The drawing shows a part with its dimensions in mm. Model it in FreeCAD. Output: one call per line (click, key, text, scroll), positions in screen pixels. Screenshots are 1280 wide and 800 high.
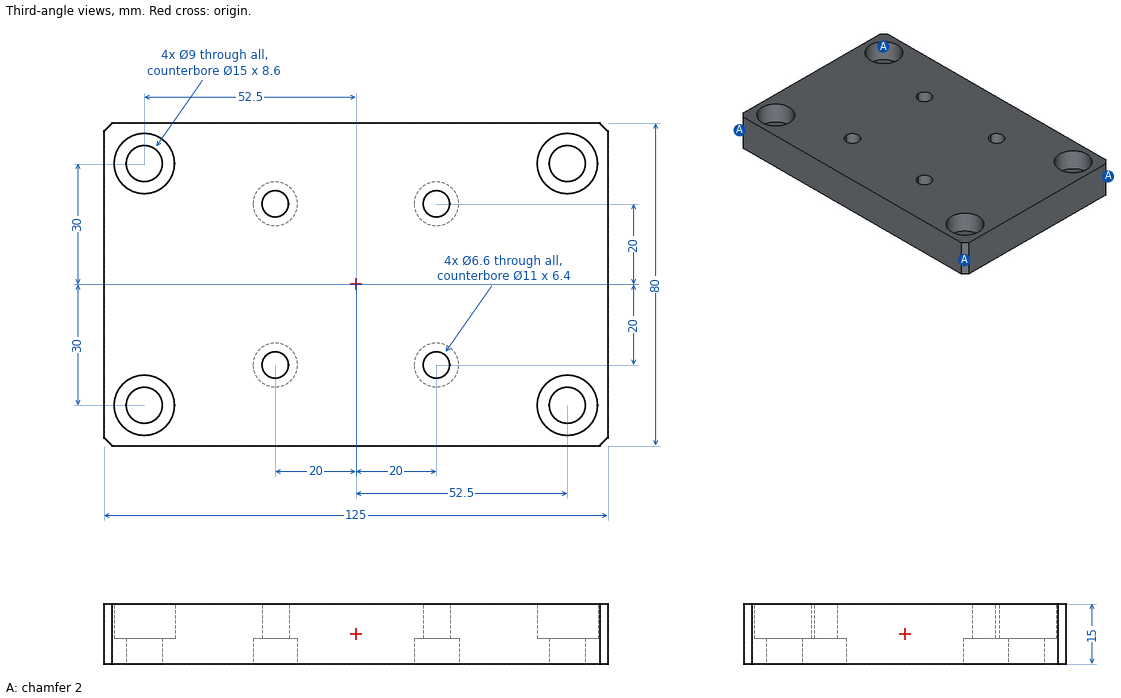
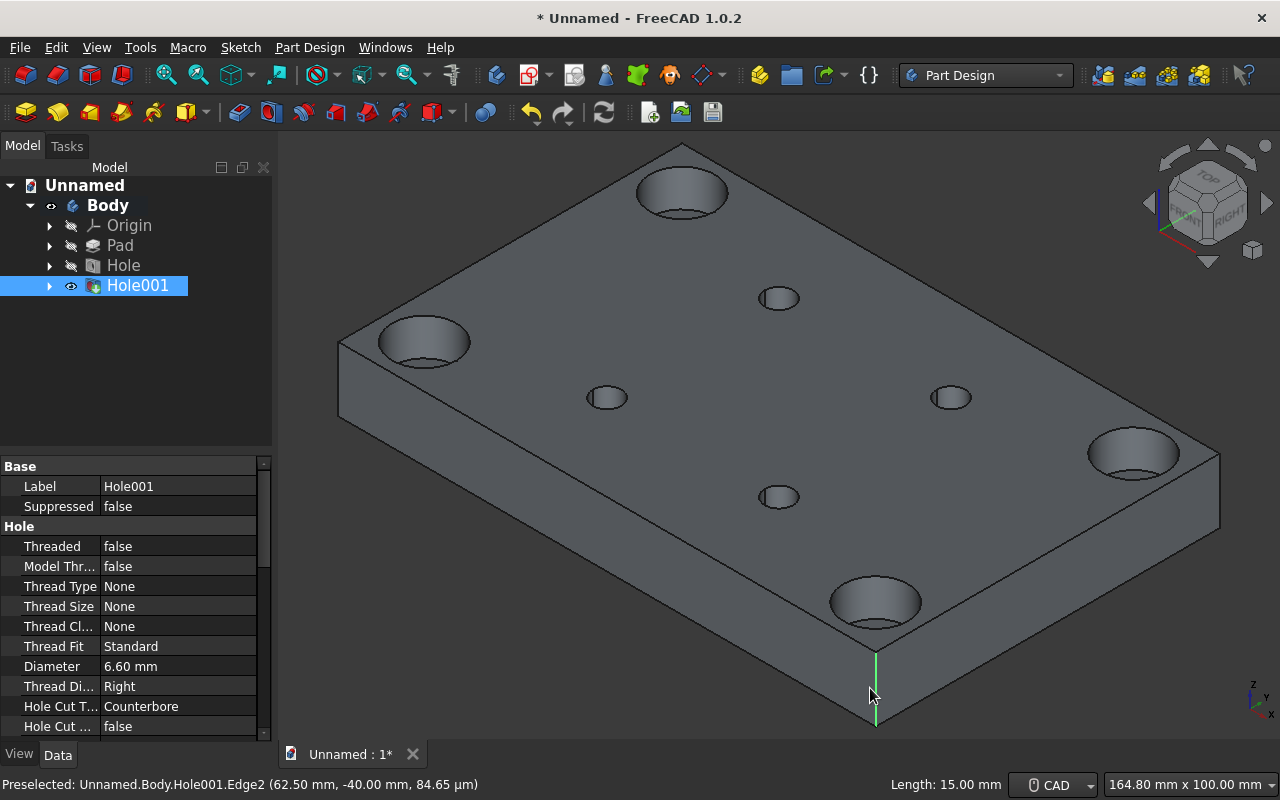
key(2)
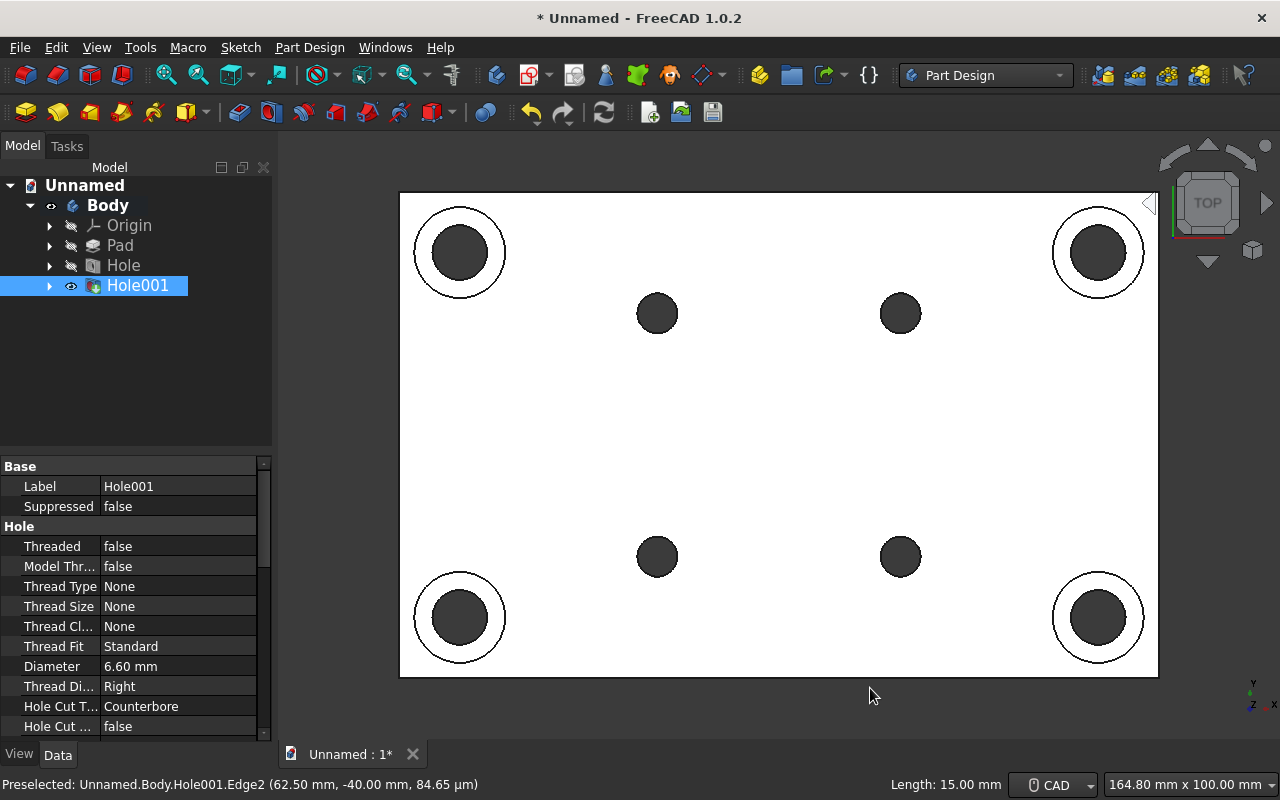
key(1)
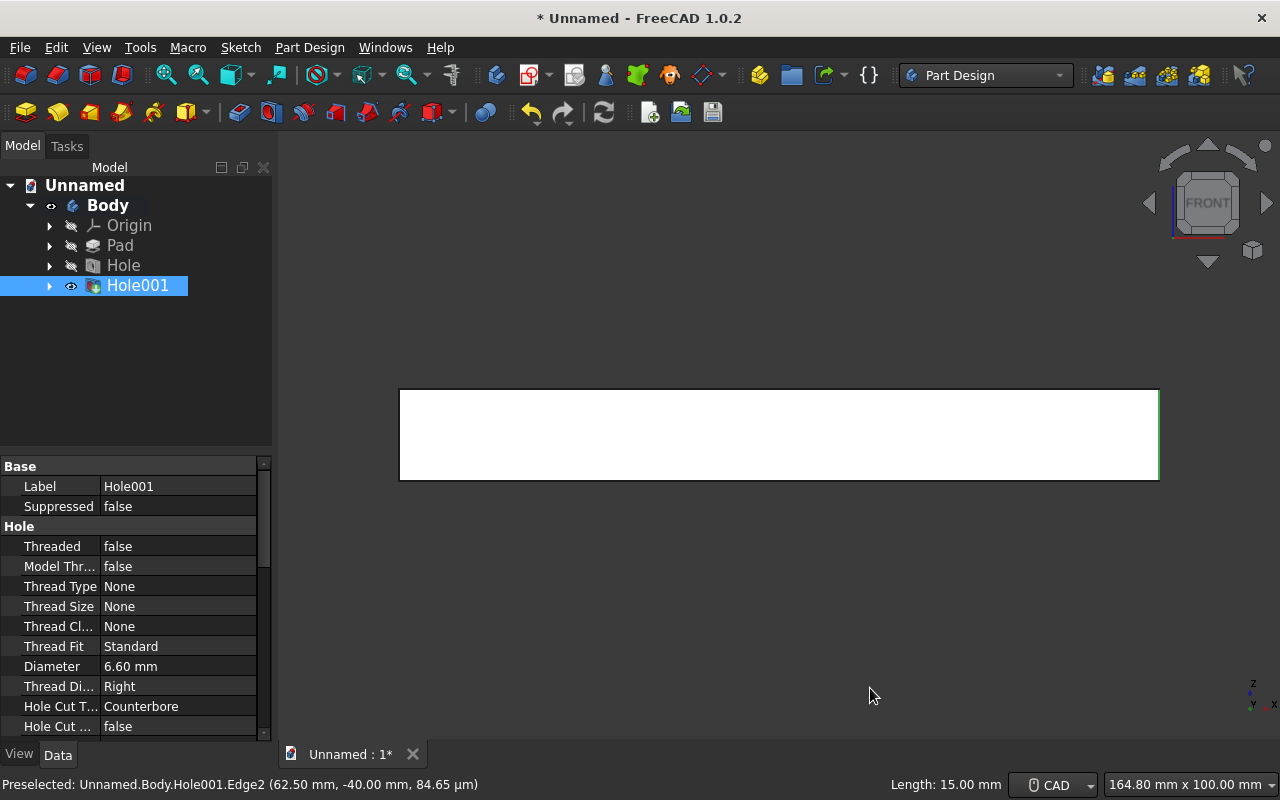
click(399, 434, ctrl)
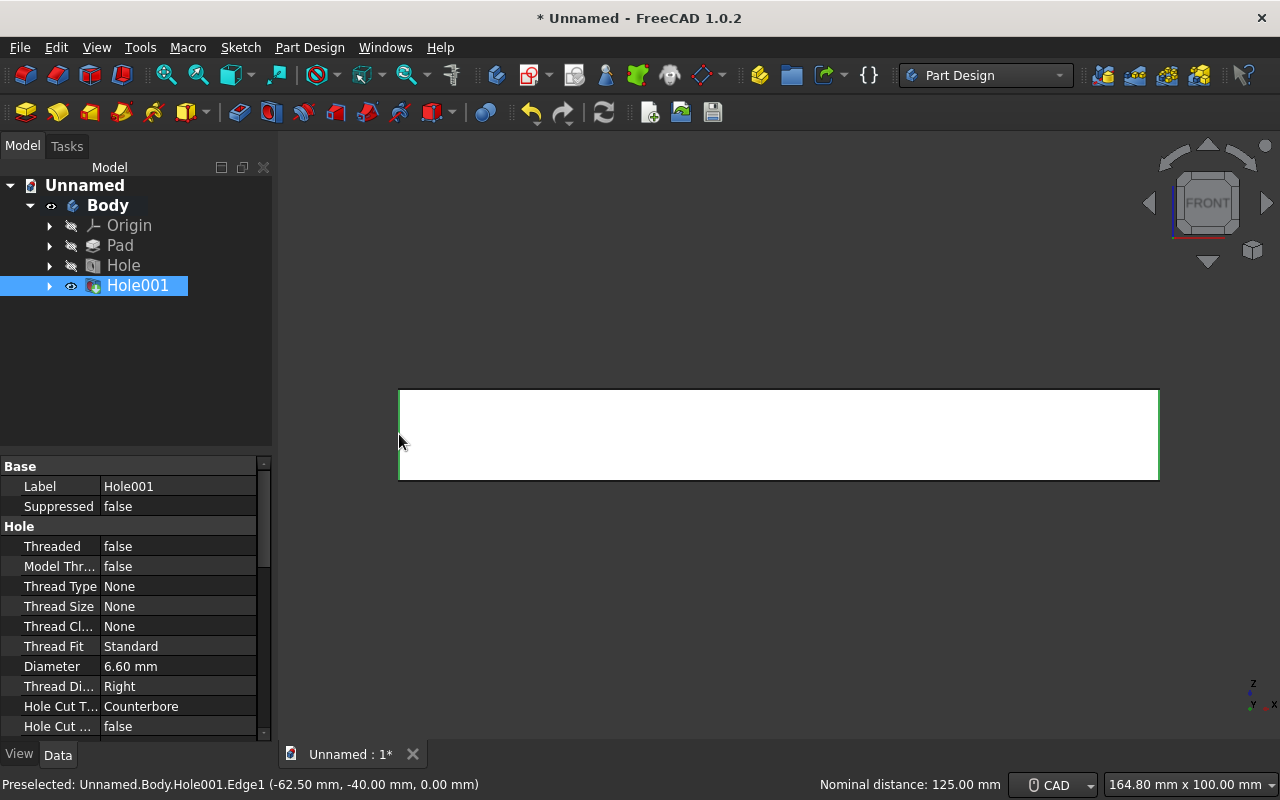
key(3)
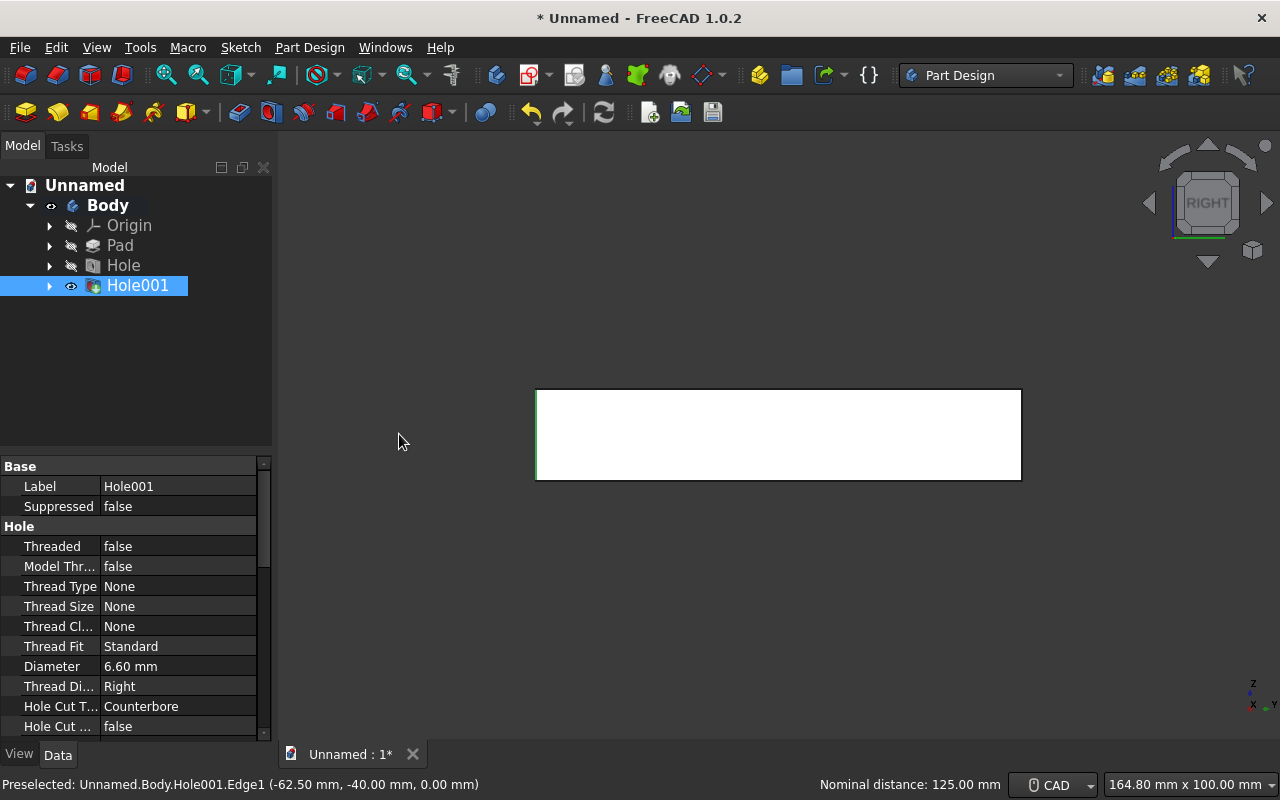
click(1022, 434, ctrl)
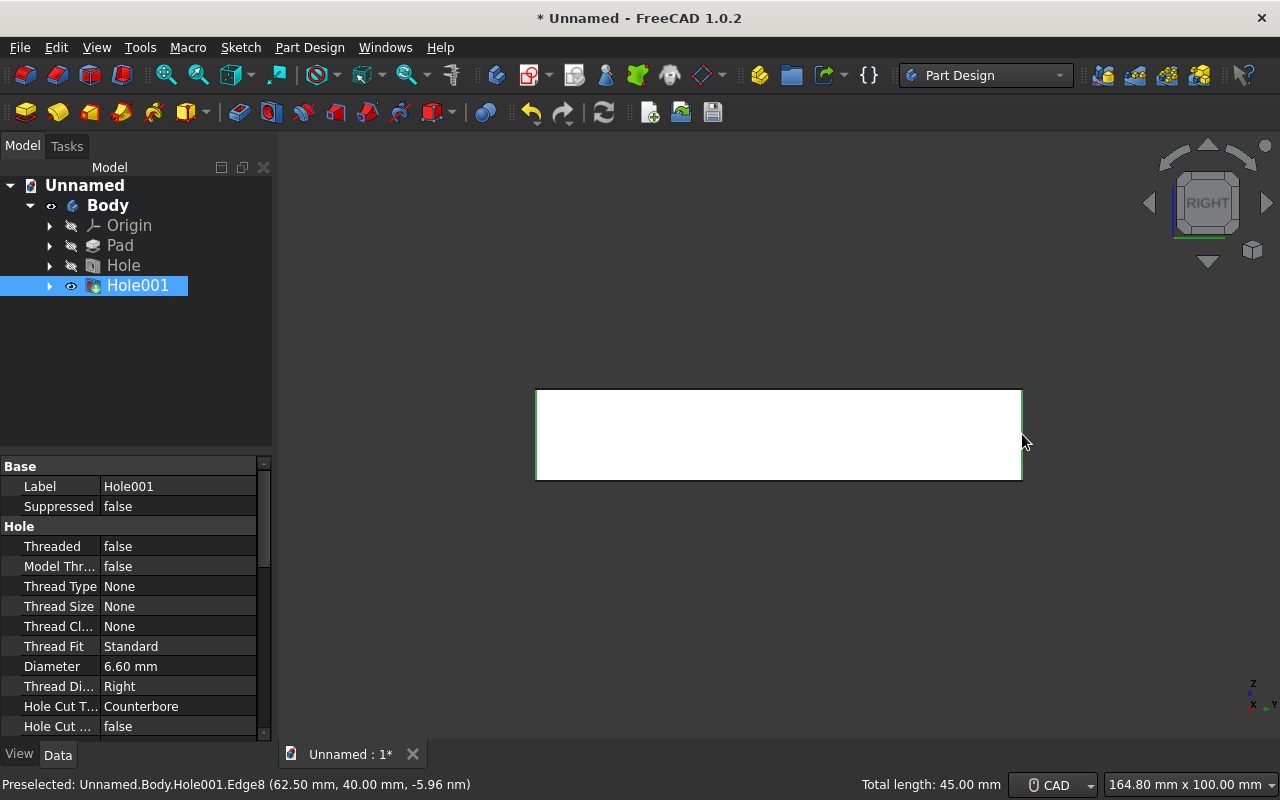
key(5)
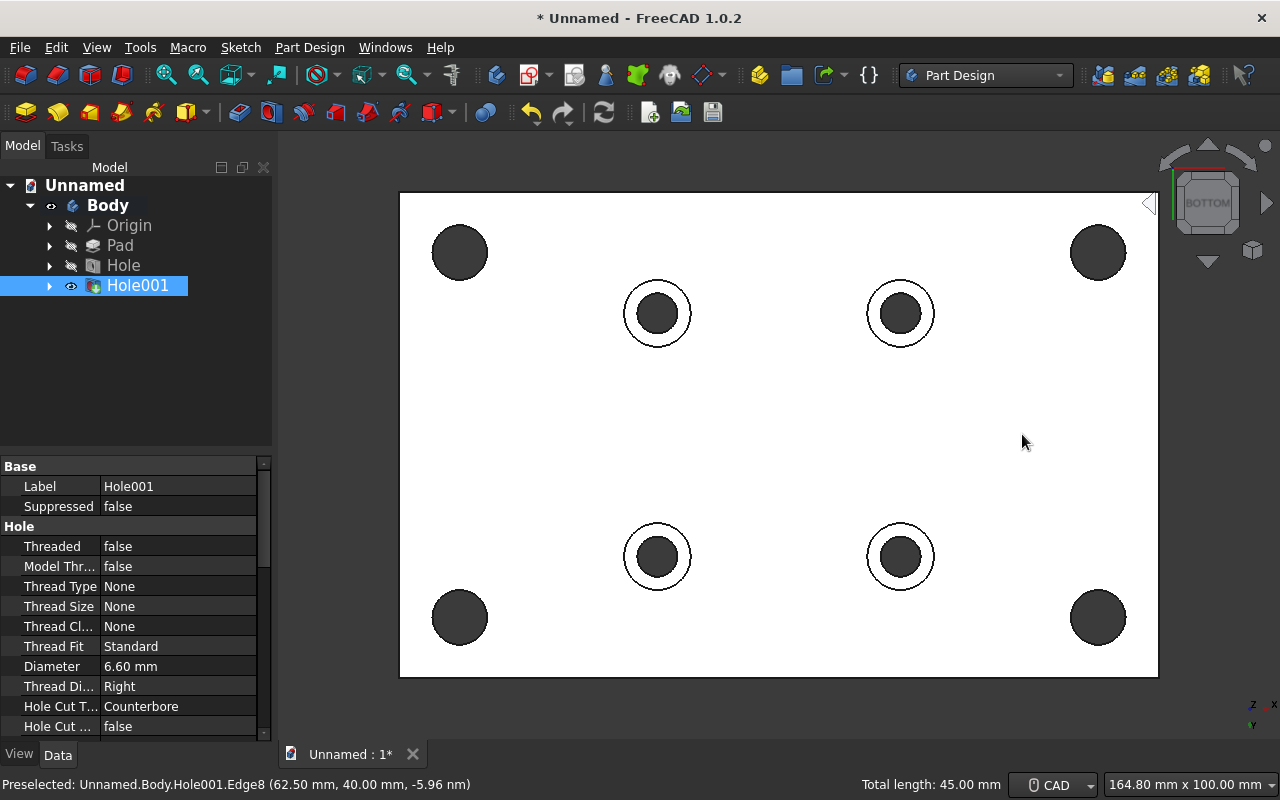
key(4)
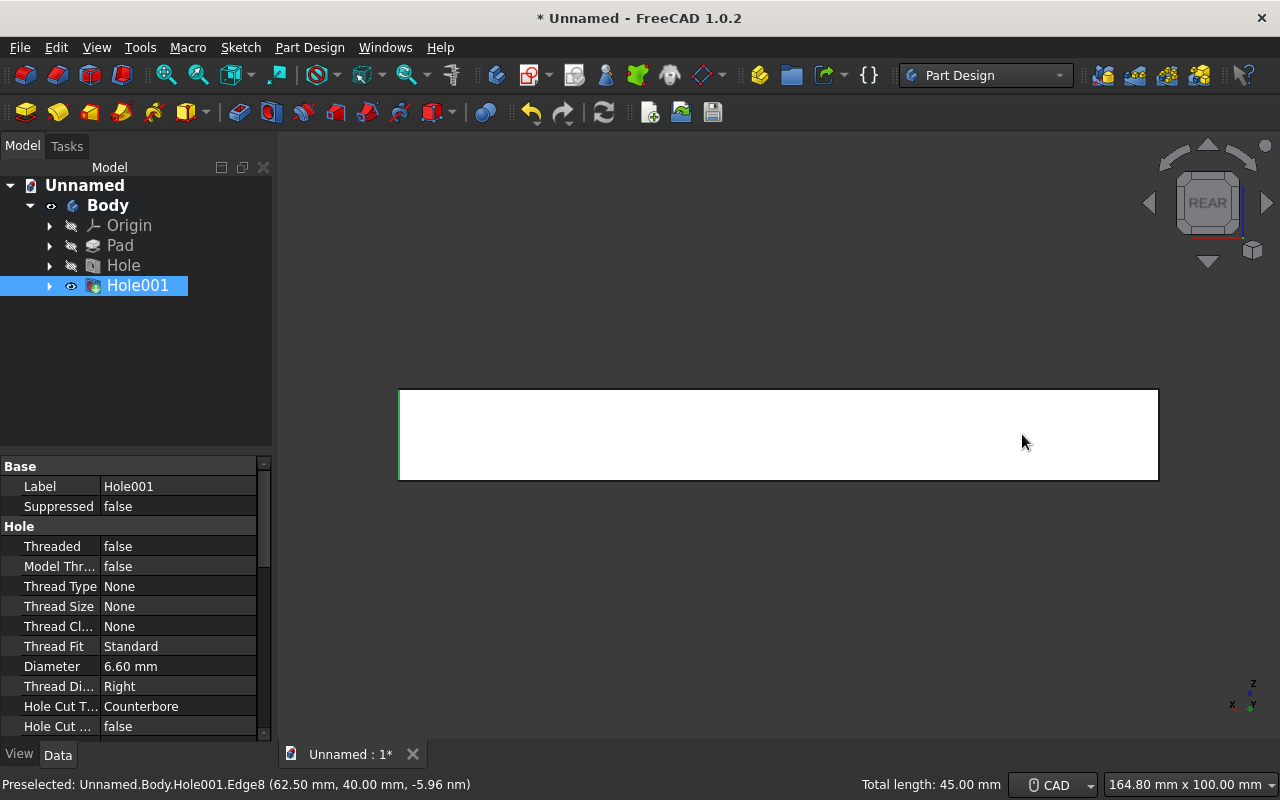
click(1159, 434, ctrl)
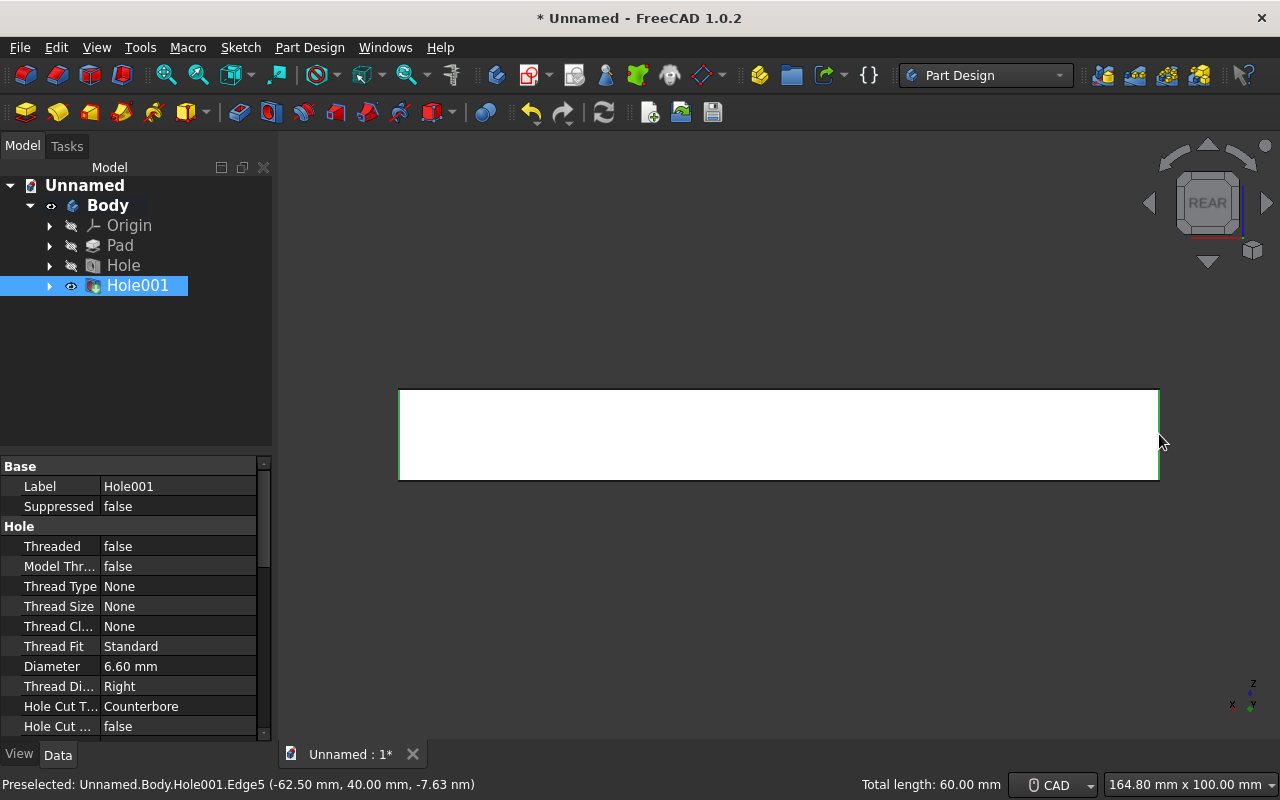
click(58, 76)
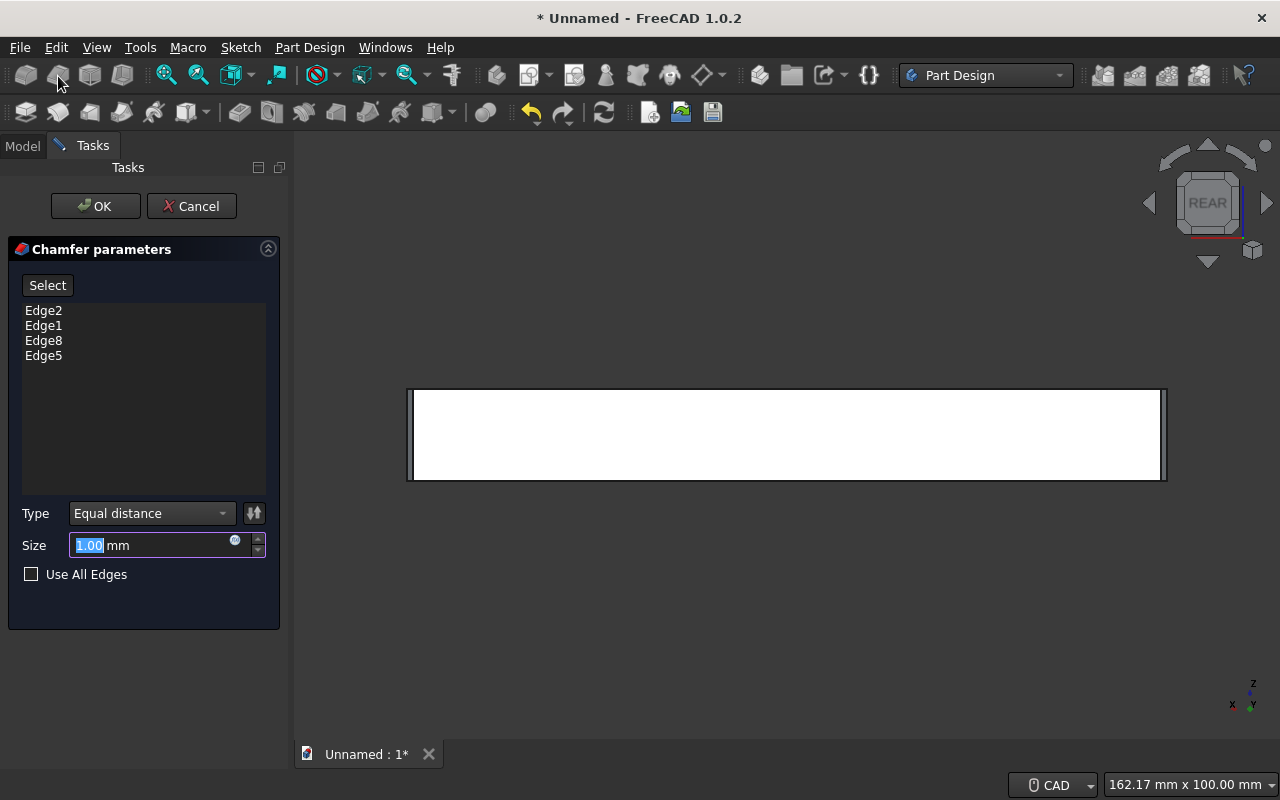
text(2)
key(Tab)